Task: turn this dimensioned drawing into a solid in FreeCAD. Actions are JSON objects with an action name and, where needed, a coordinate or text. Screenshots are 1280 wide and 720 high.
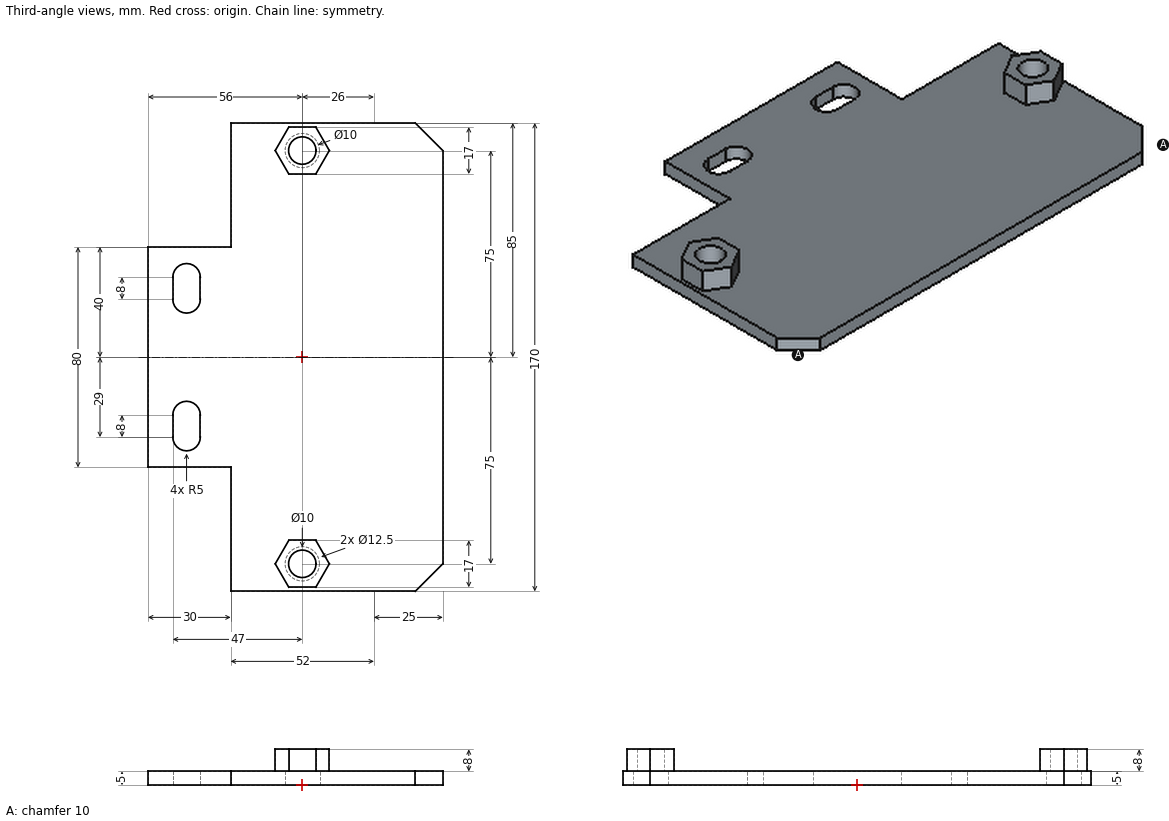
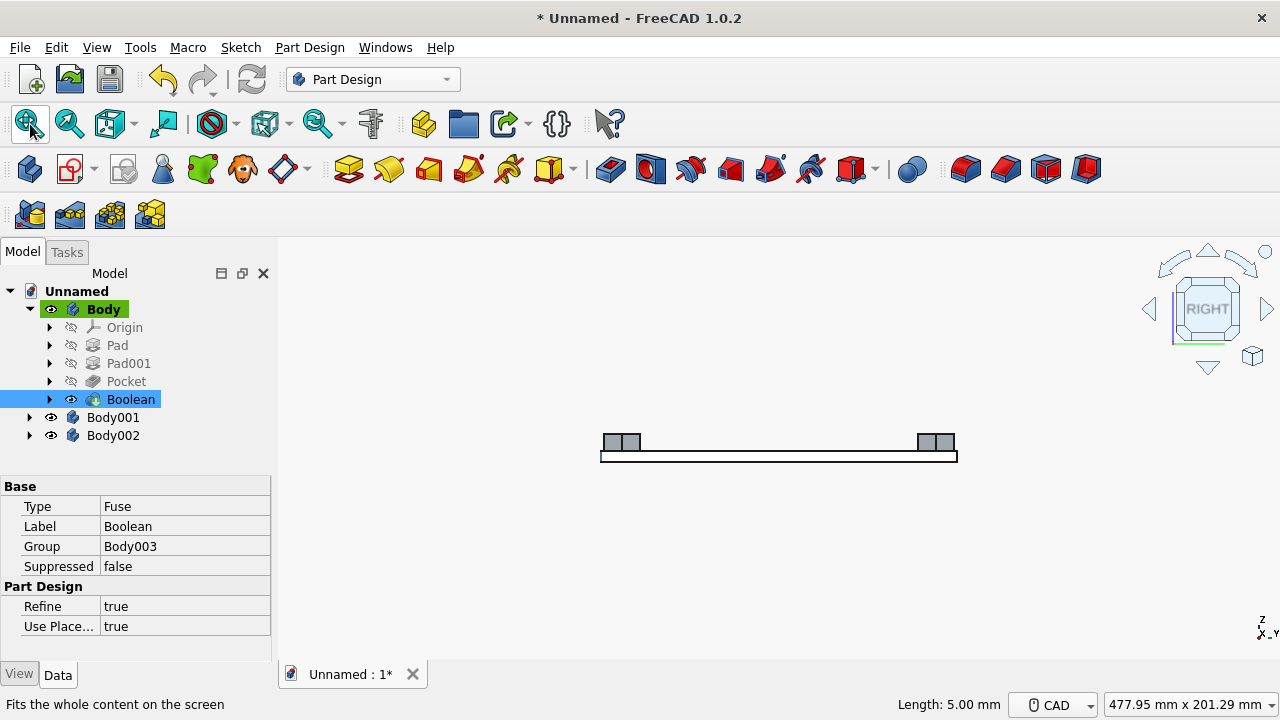
{"action": "left_click", "coordinate": [30, 124]}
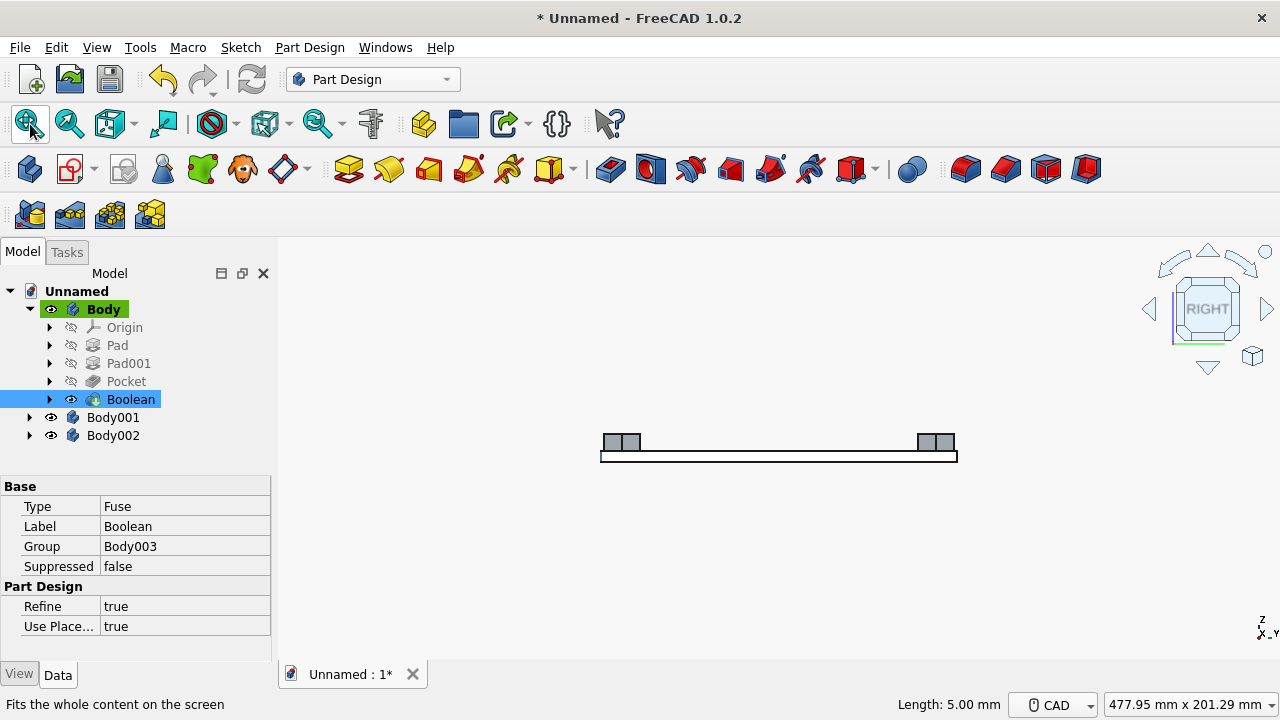
{"action": "scroll", "coordinate": [957, 455], "scroll_direction": "up", "scroll_amount": 7}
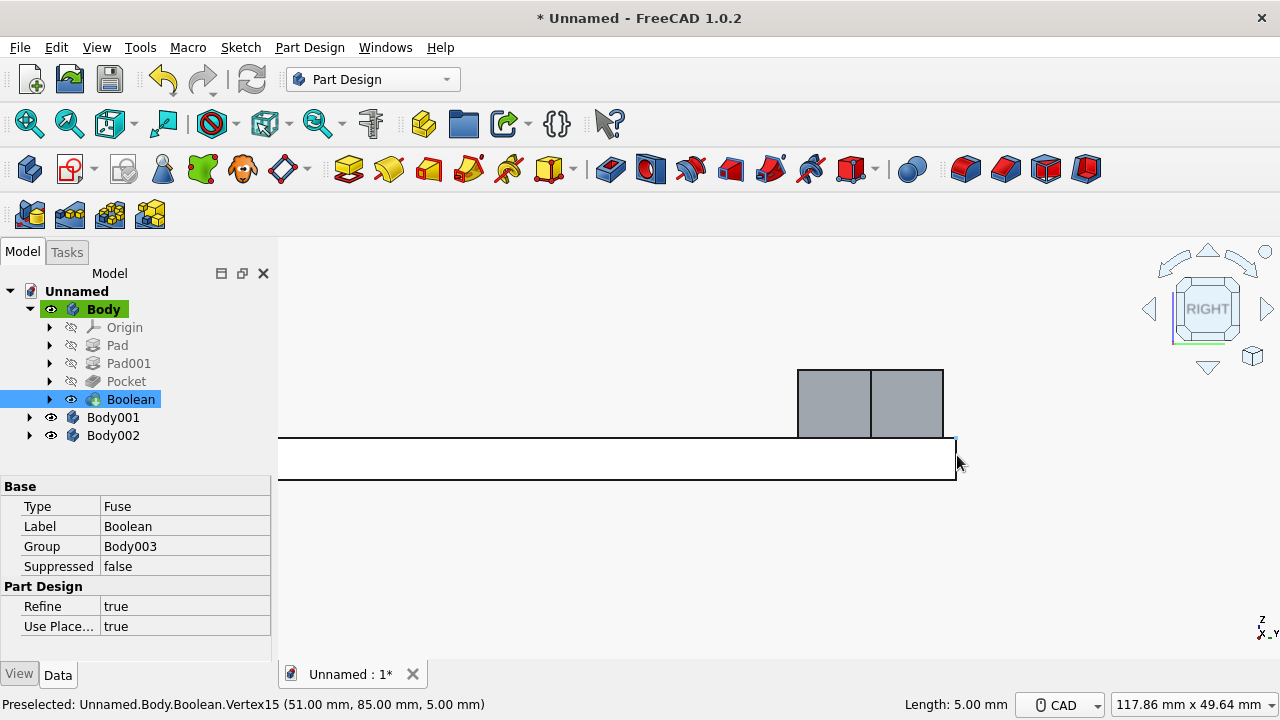
{"action": "left_click", "coordinate": [956, 458], "text": "ctrl"}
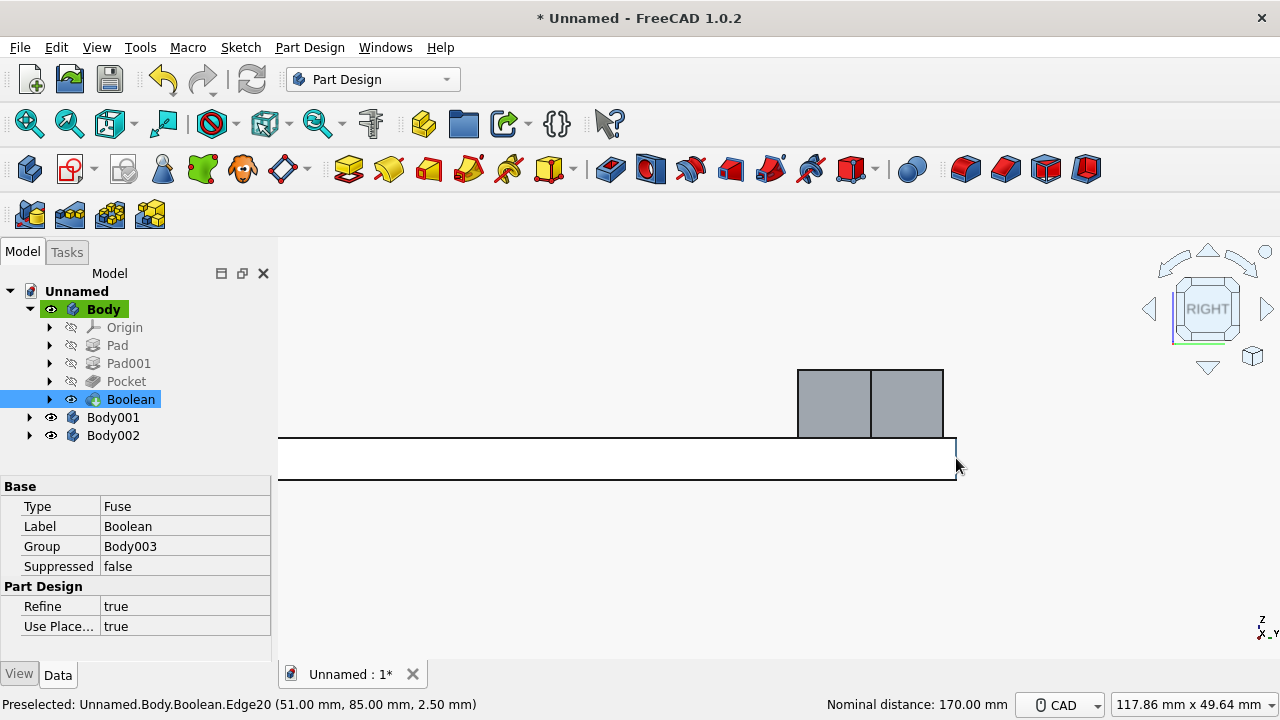
{"action": "left_click", "coordinate": [1006, 170]}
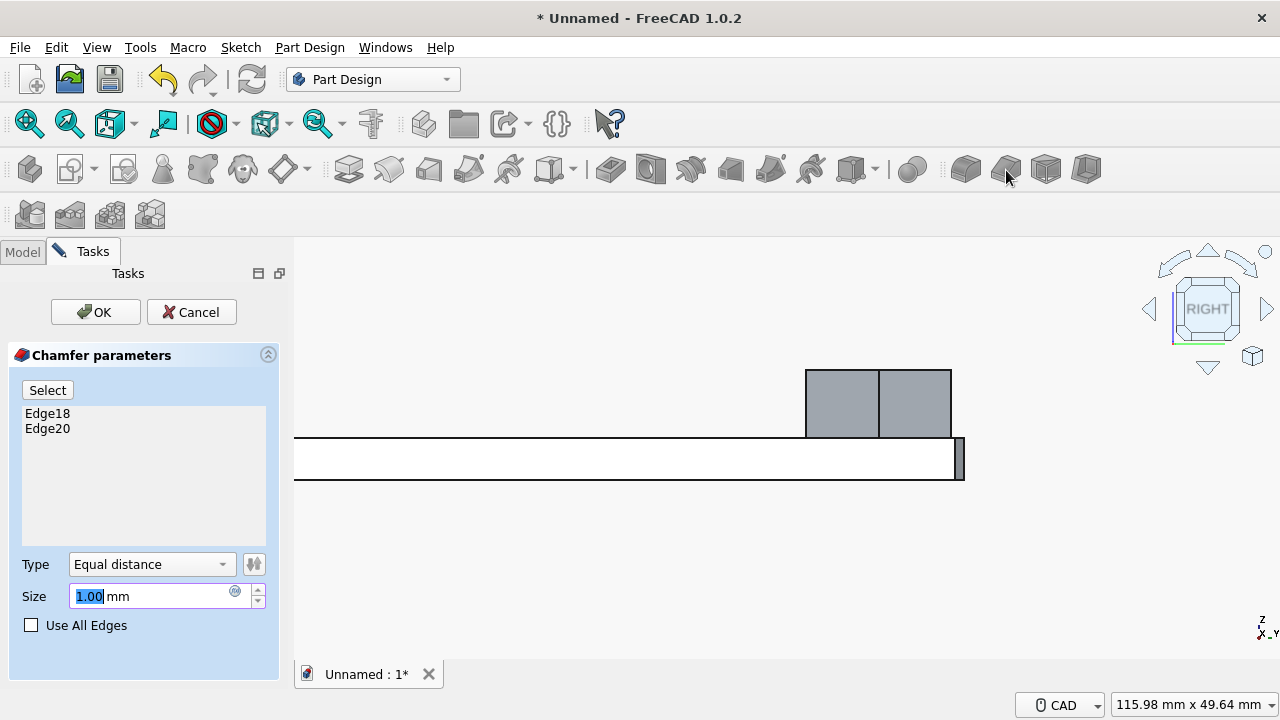
{"action": "type", "text": "10"}
{"action": "key", "text": "Tab"}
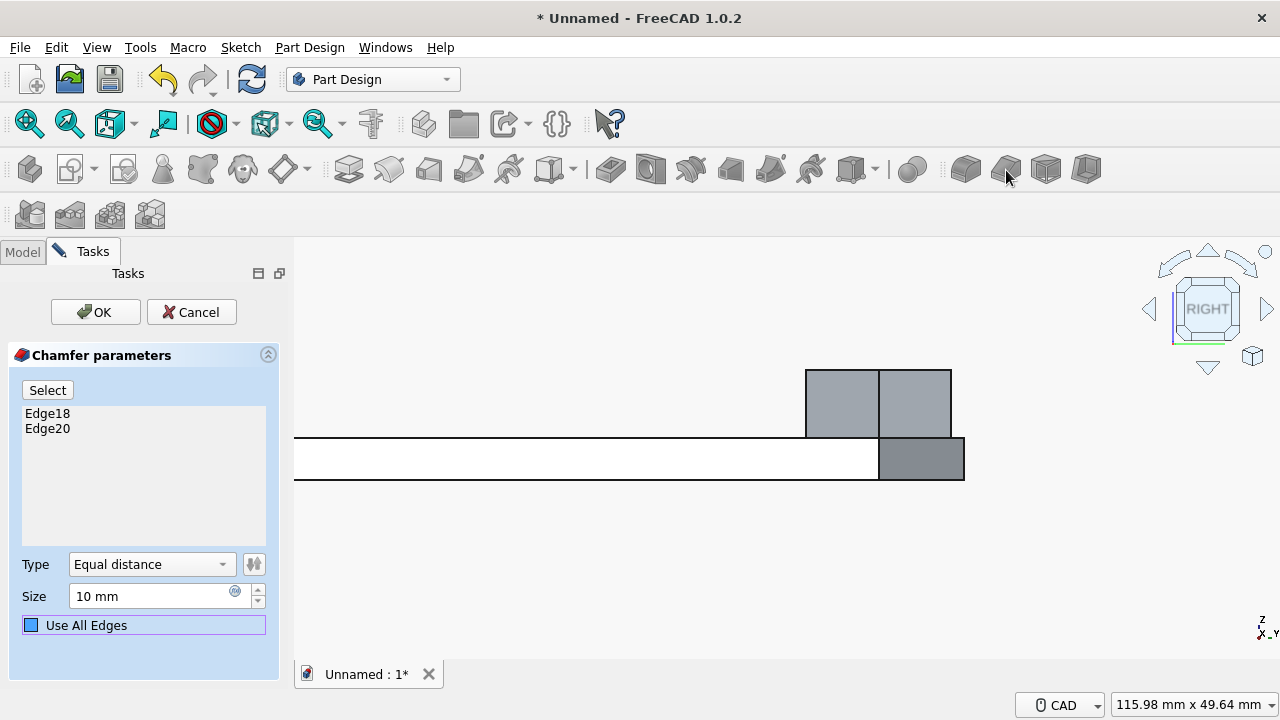
{"action": "left_click", "coordinate": [96, 312]}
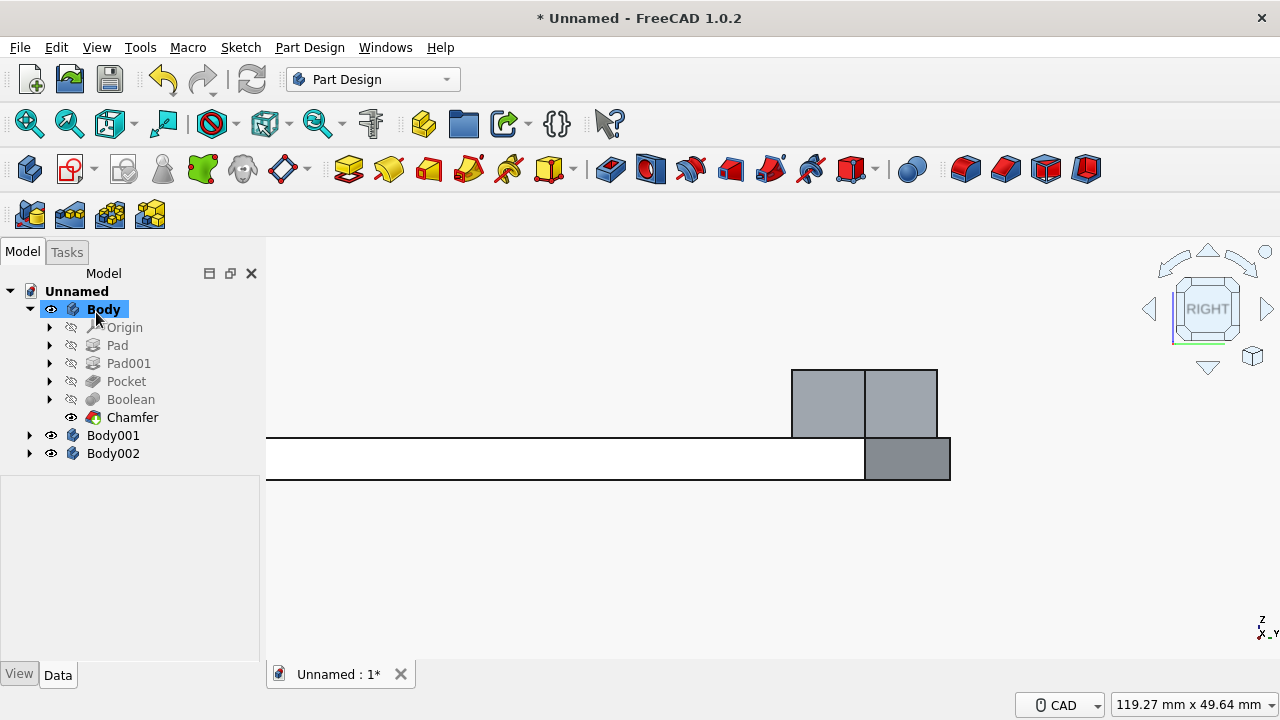
{"action": "key", "text": "0"}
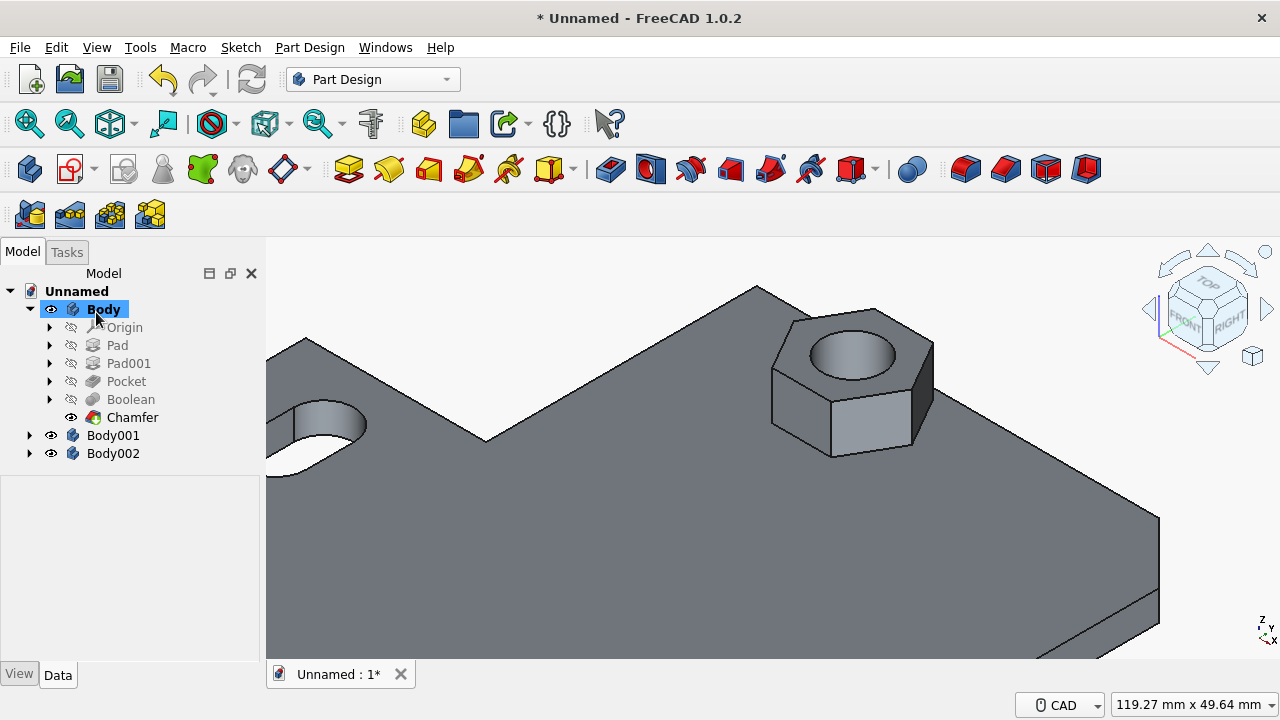
{"action": "left_click", "coordinate": [30, 124]}